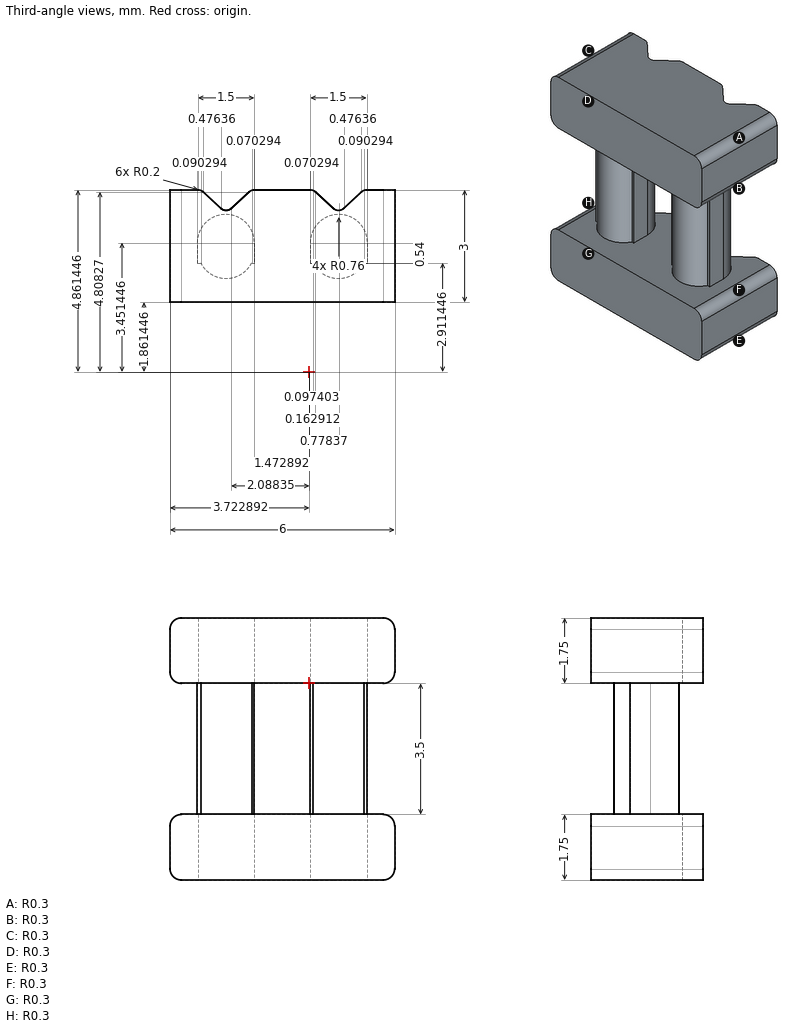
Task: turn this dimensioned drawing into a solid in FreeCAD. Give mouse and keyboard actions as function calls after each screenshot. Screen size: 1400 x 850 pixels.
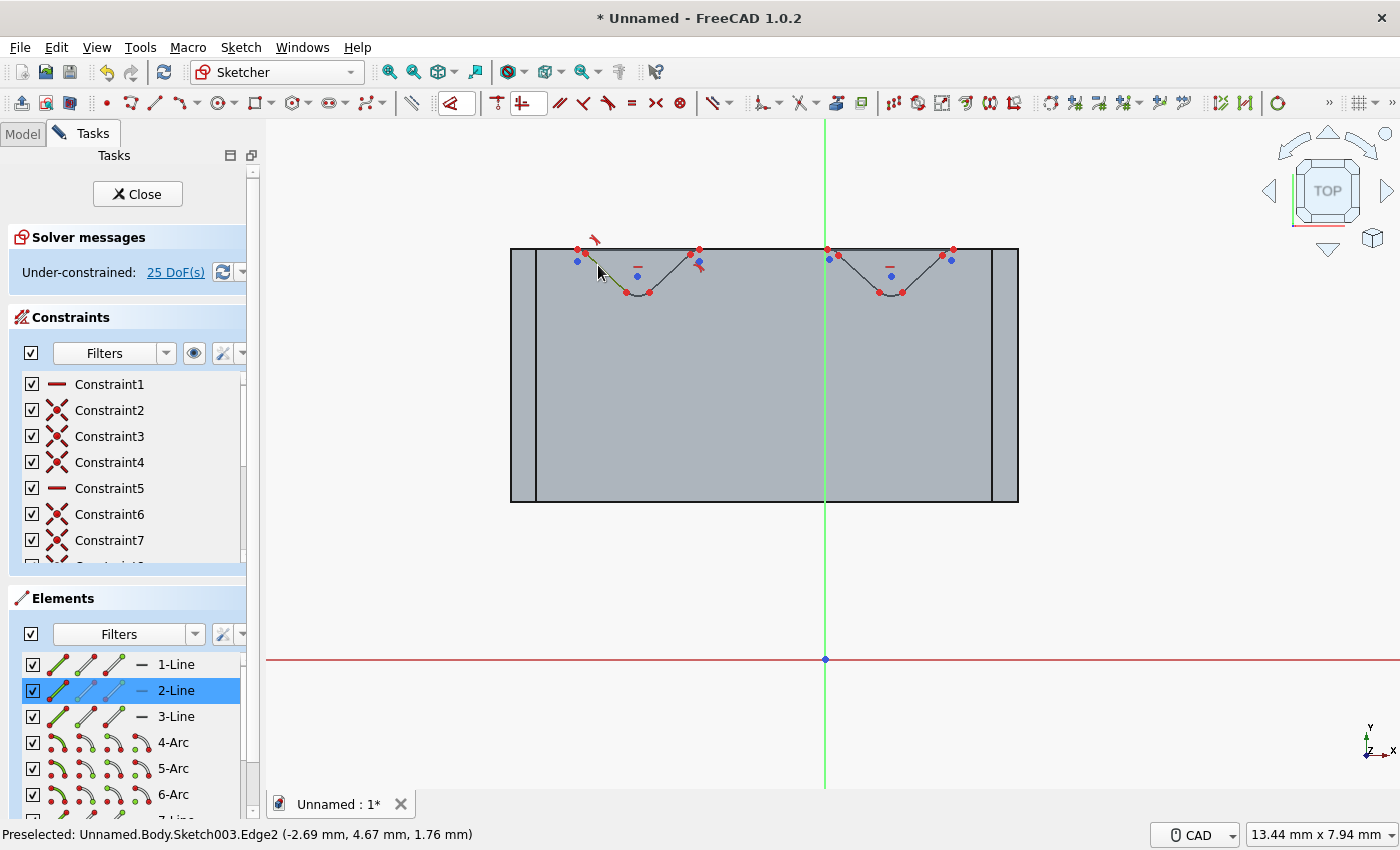
click(638, 296)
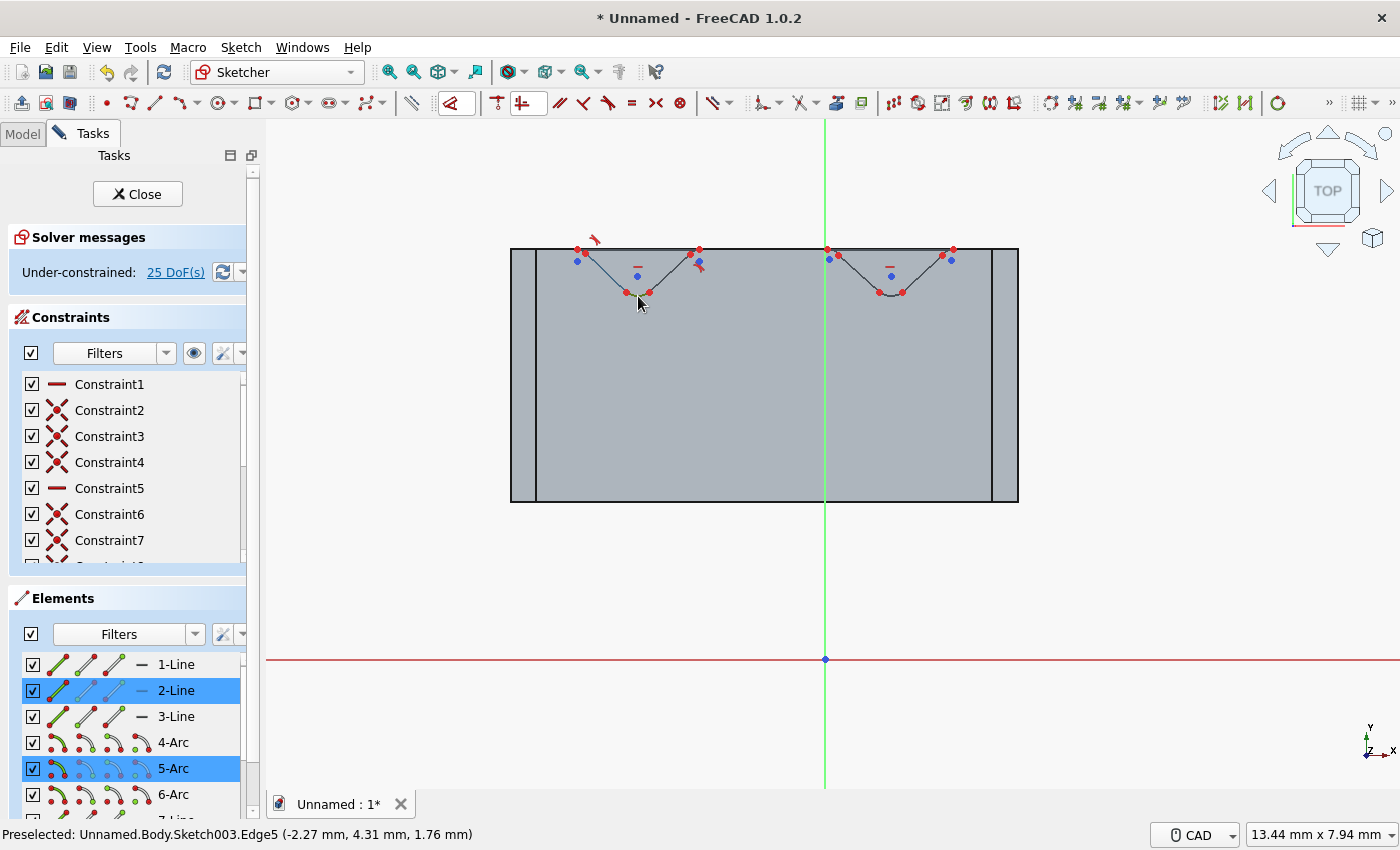
click(608, 104)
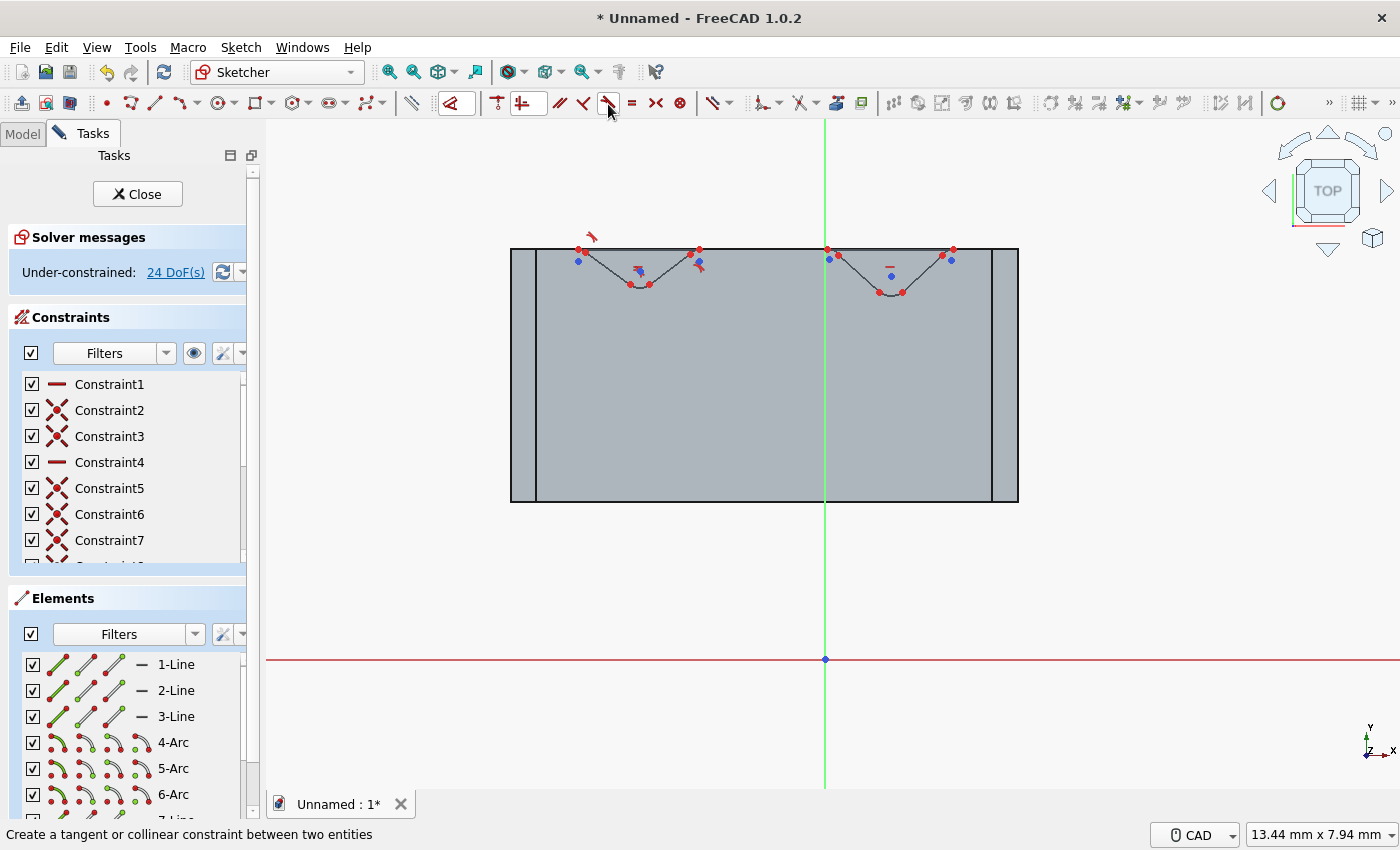
click(662, 276)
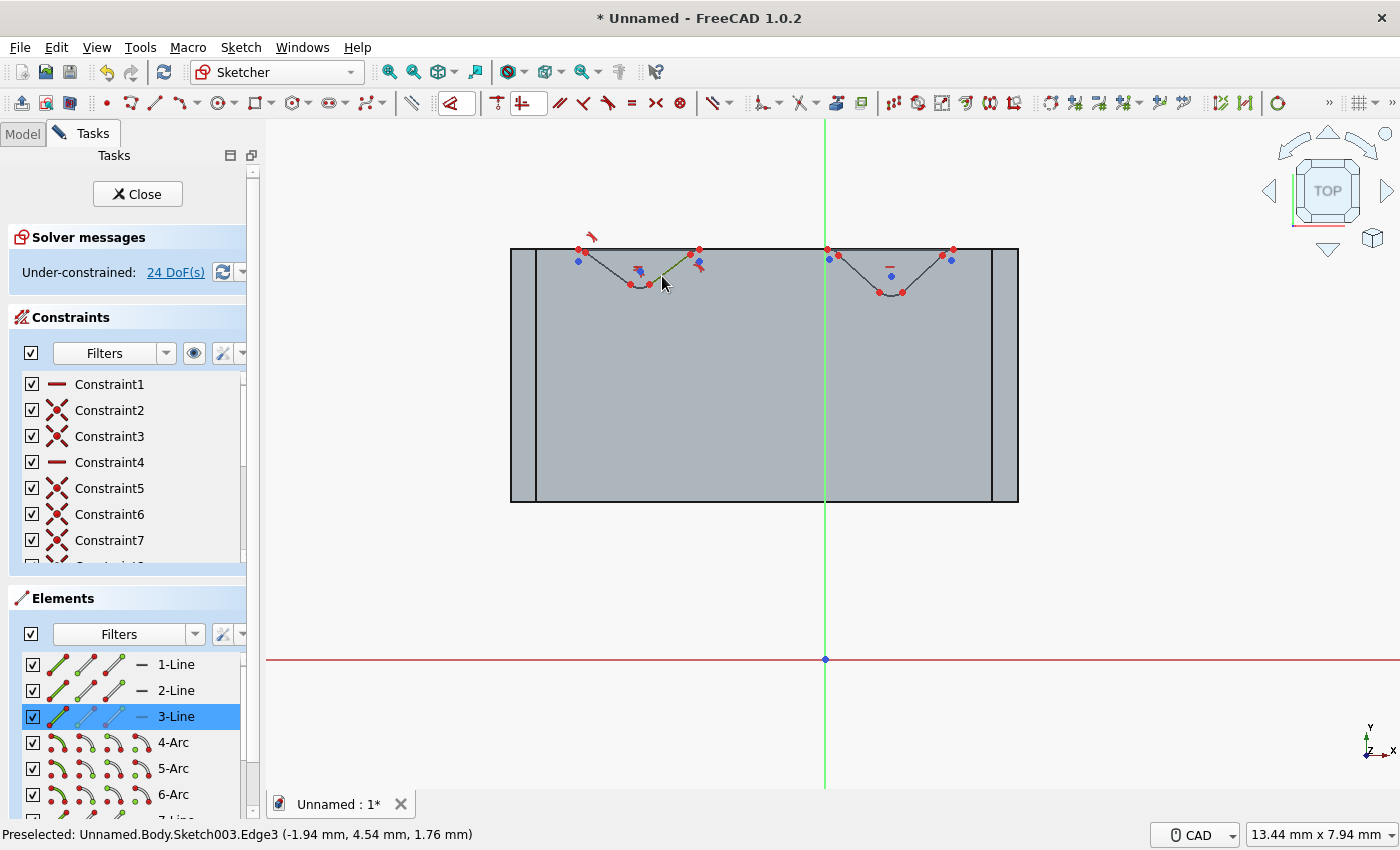
scroll(640, 288, up, 2)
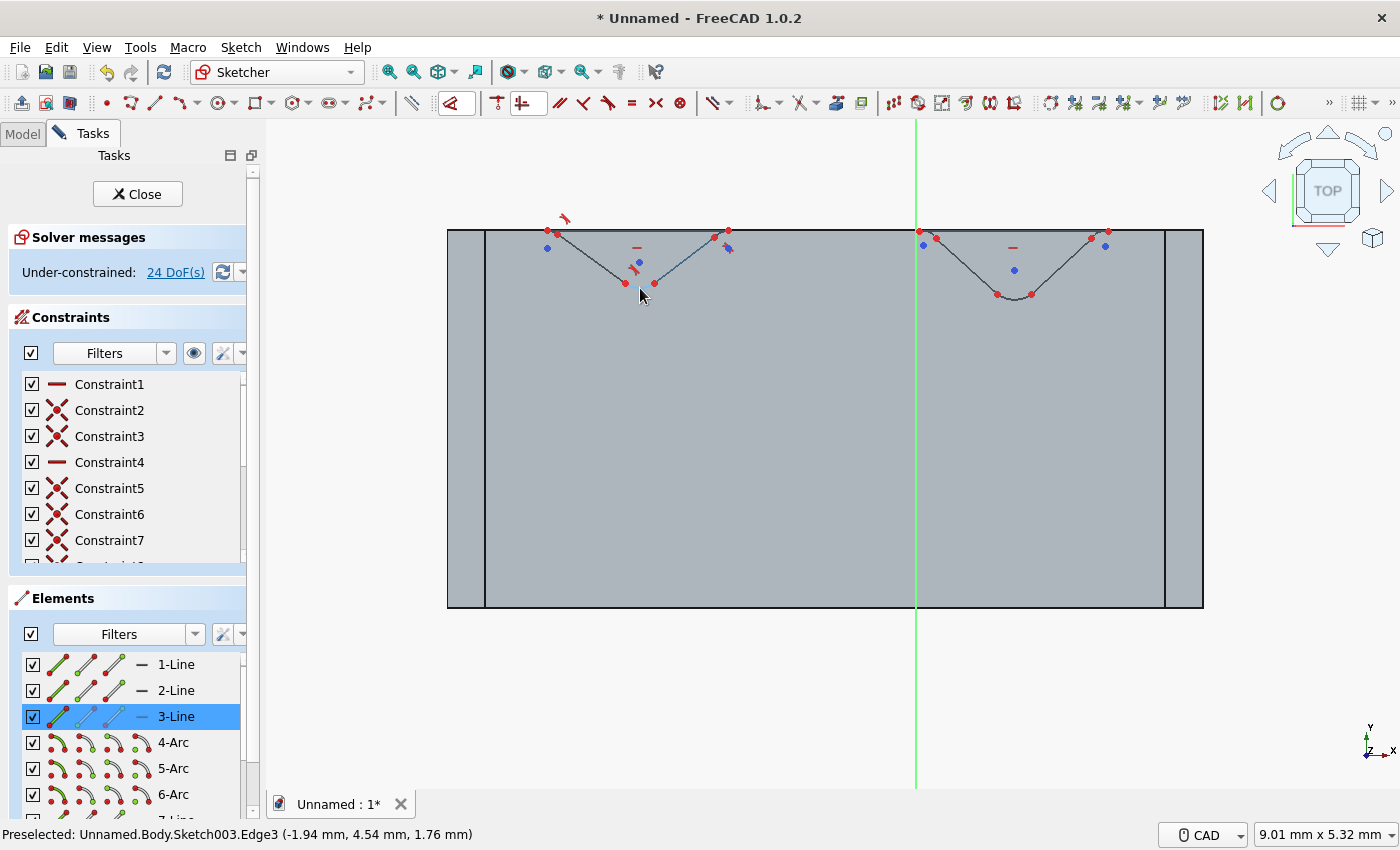
click(640, 288)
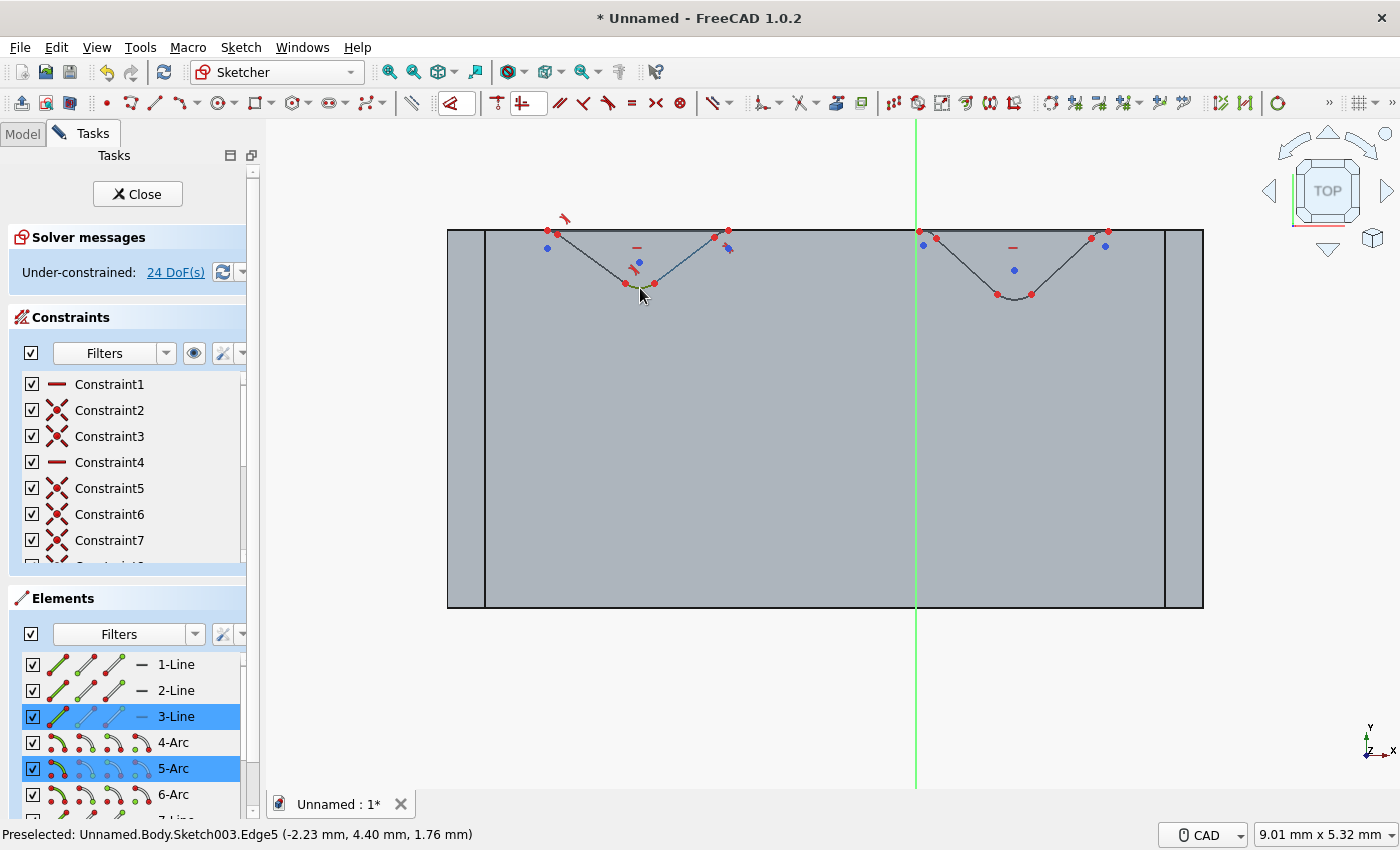
click(608, 104)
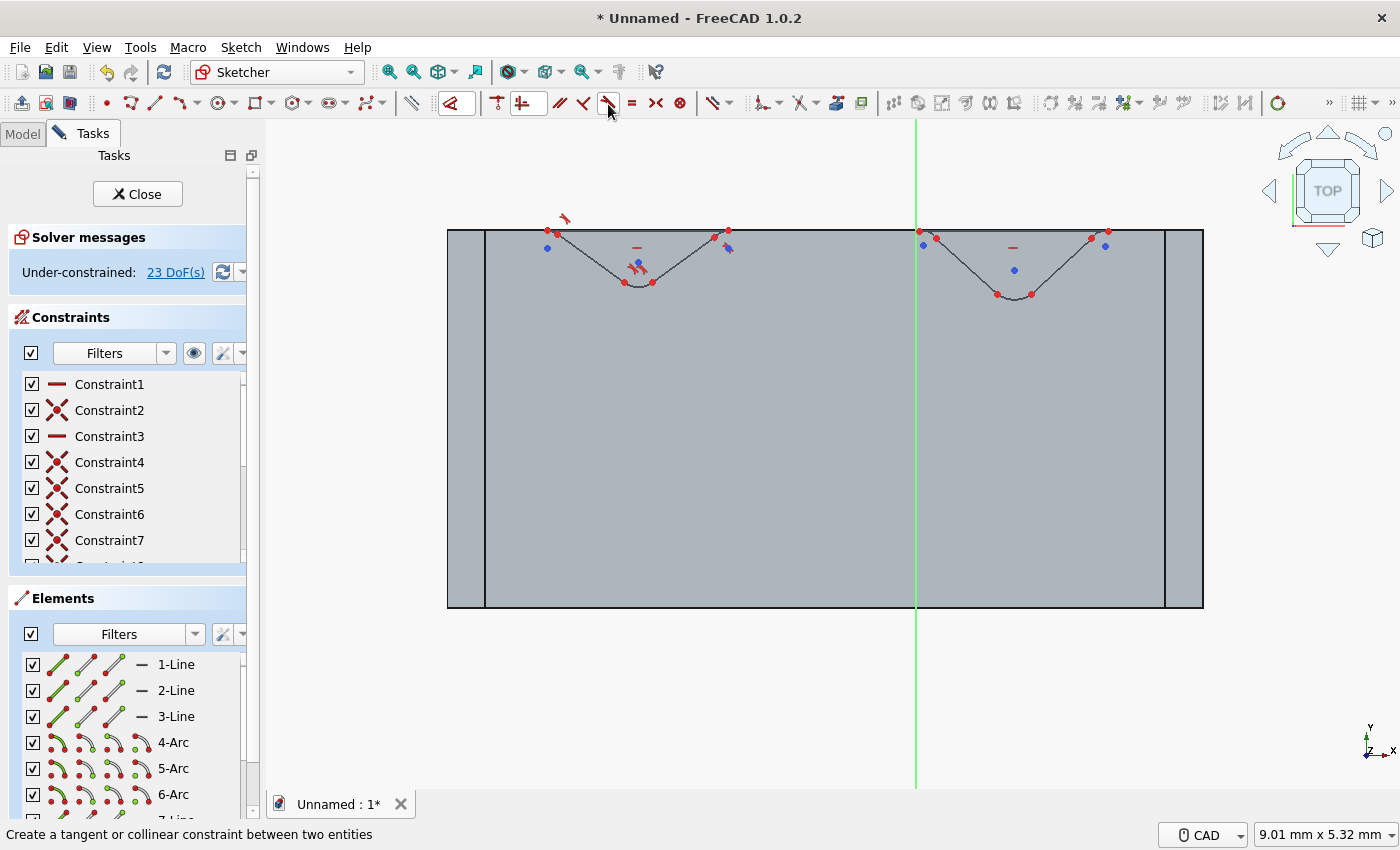
click(671, 269)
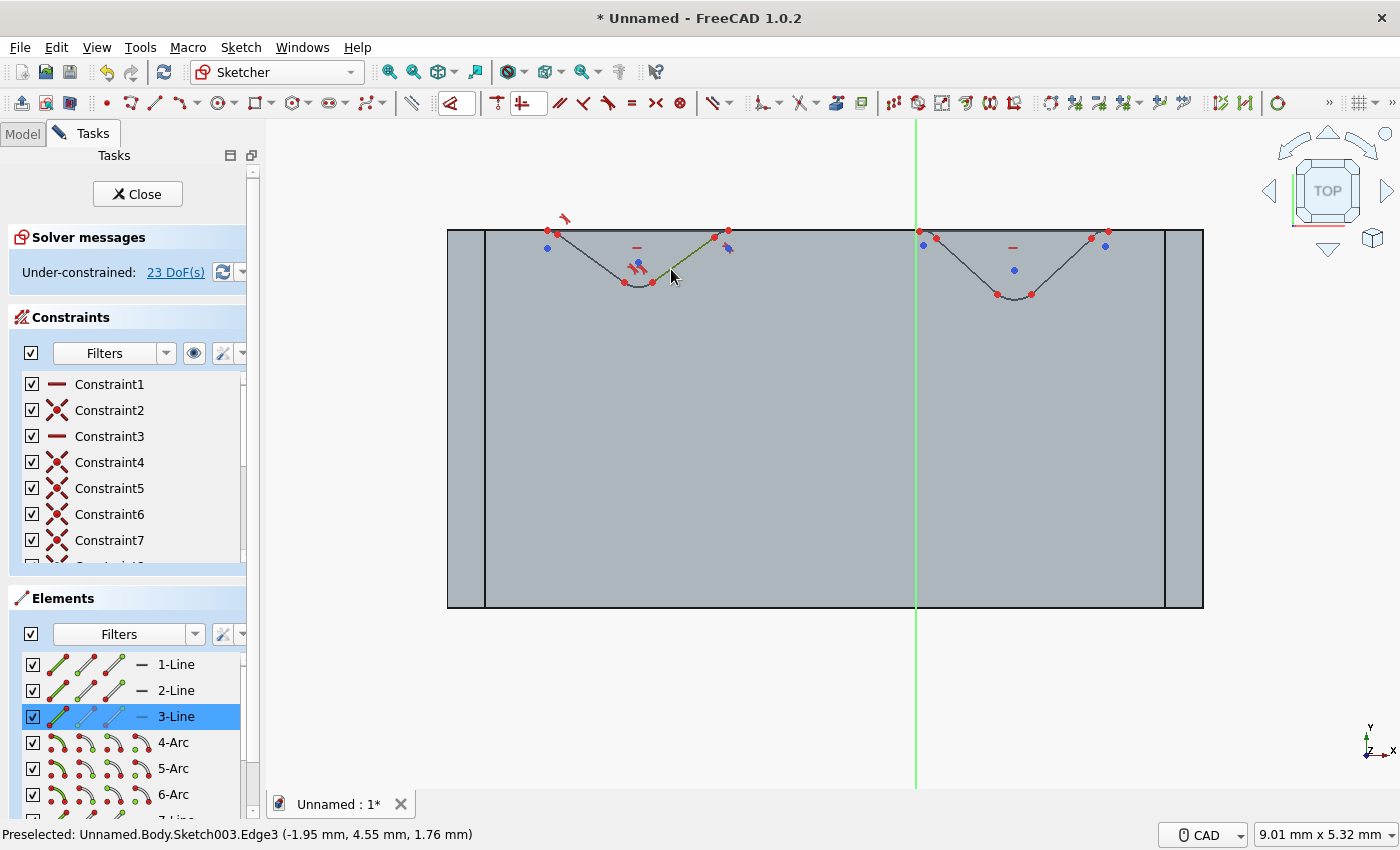
scroll(718, 234, up, 8)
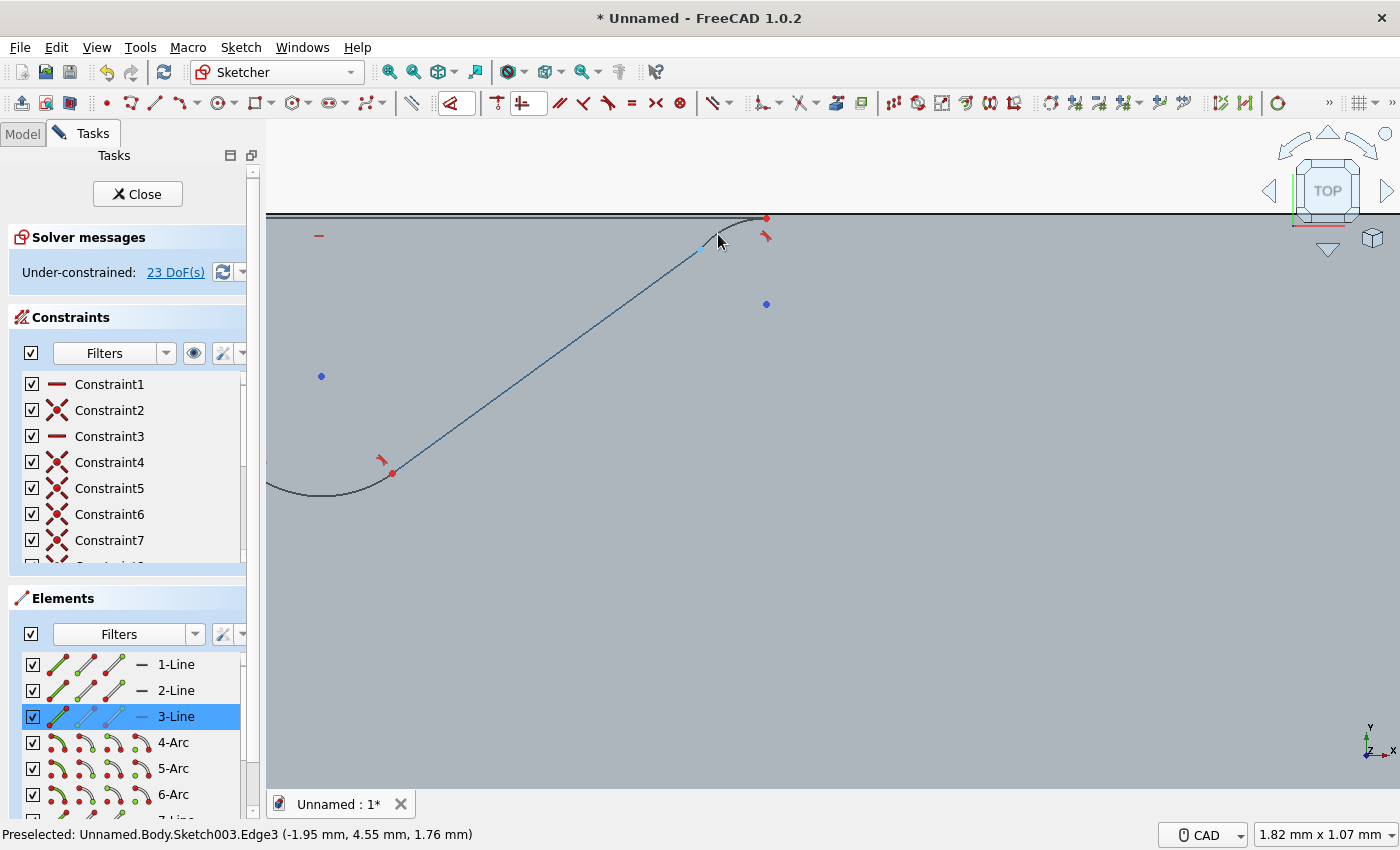
click(717, 234)